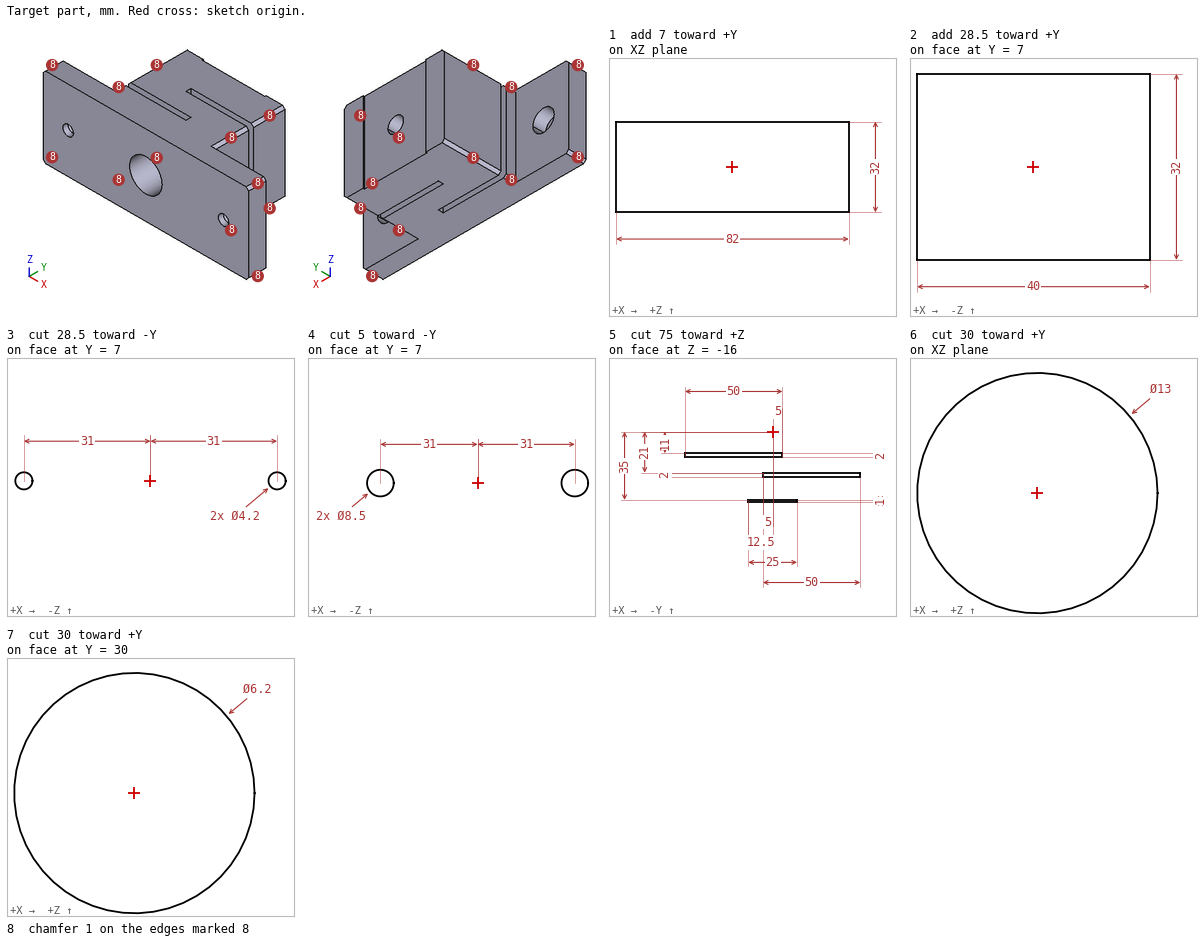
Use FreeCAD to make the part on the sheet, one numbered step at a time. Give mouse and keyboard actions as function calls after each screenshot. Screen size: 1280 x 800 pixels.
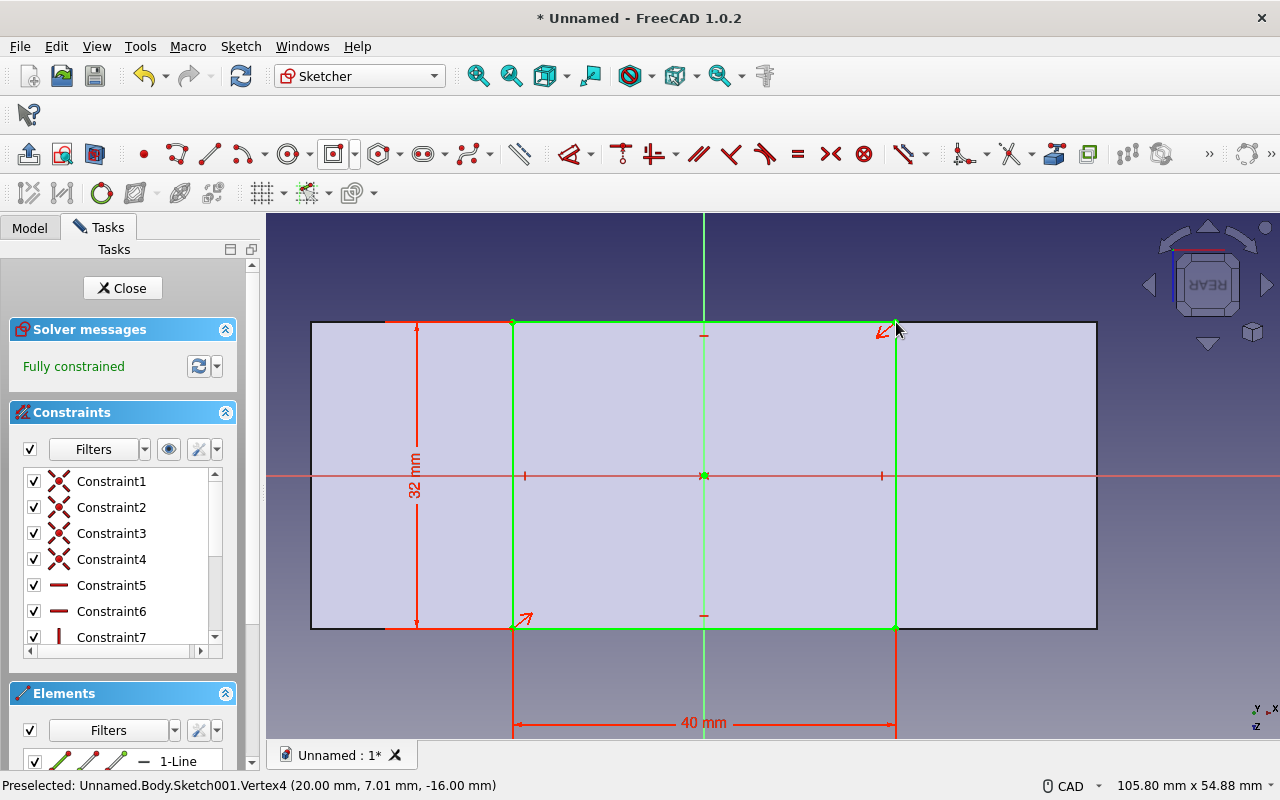
click(123, 288)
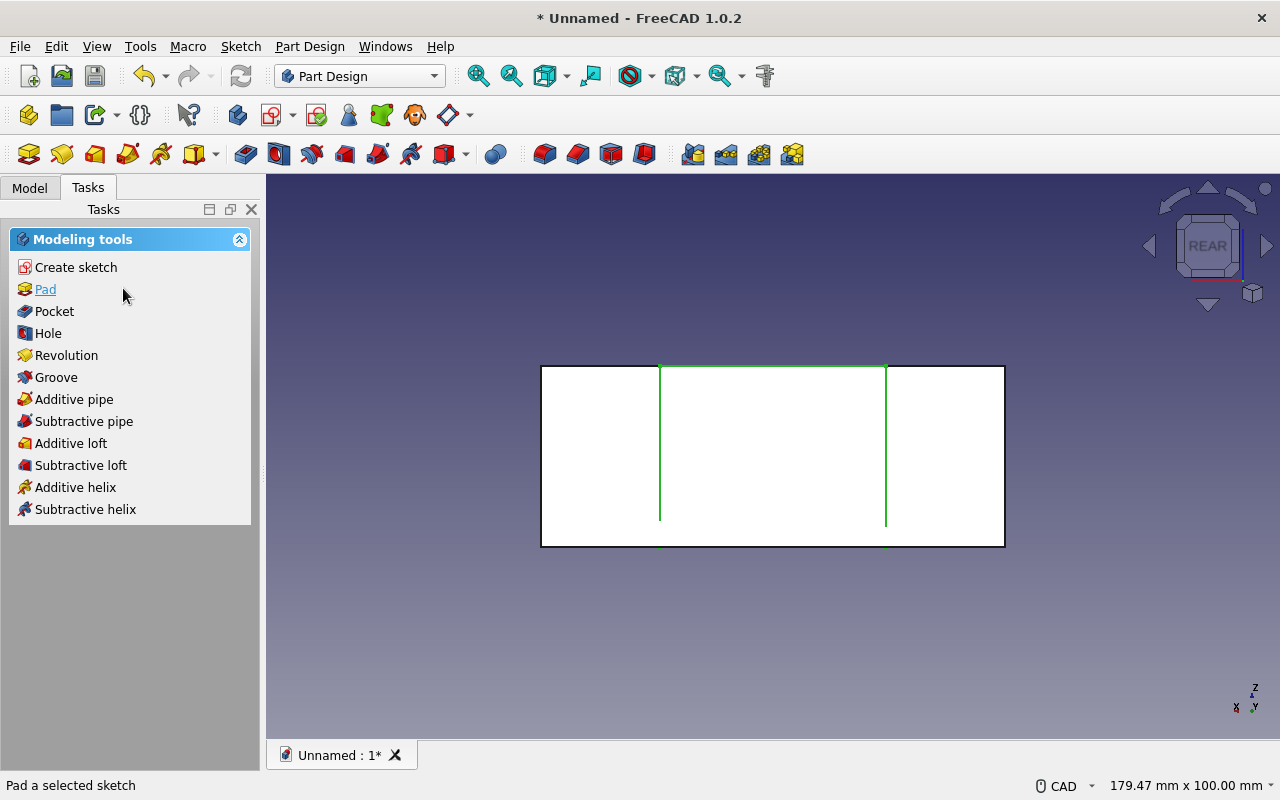
click(29, 154)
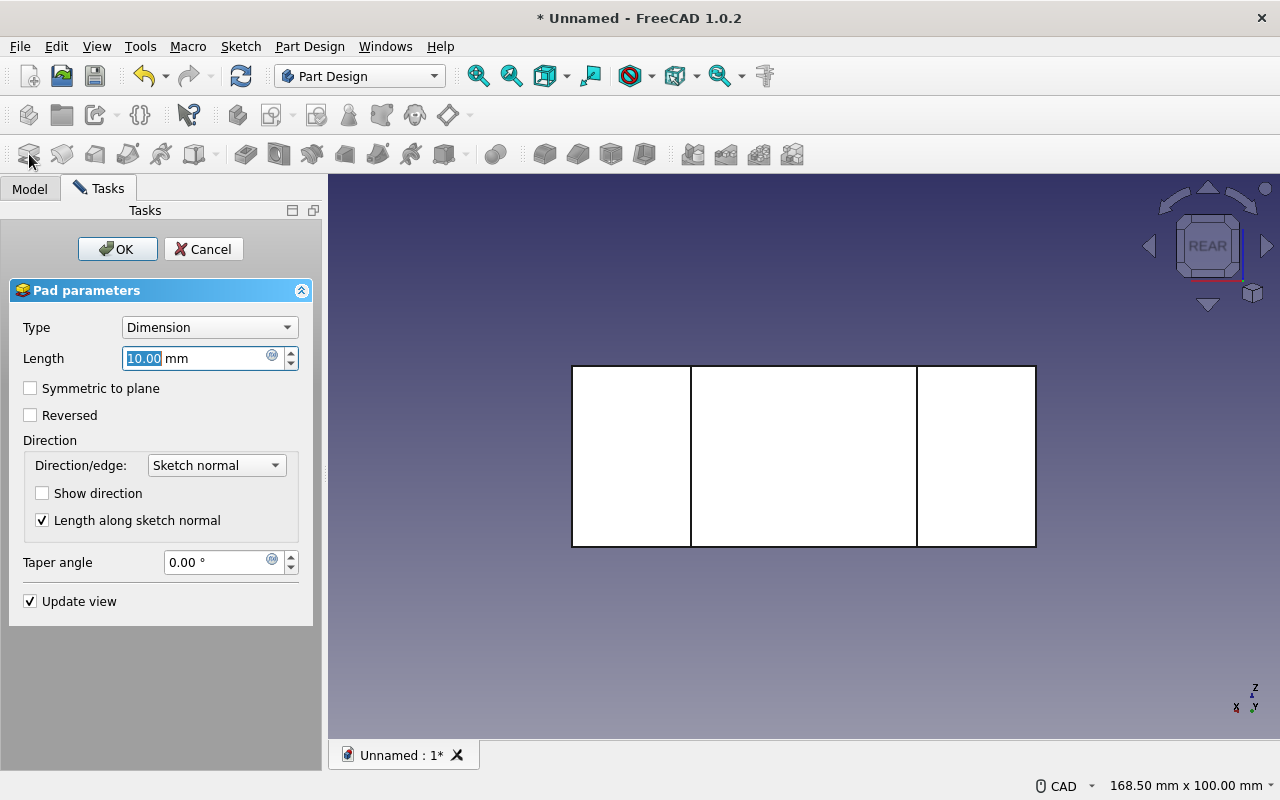
text(28.5)
key(Tab)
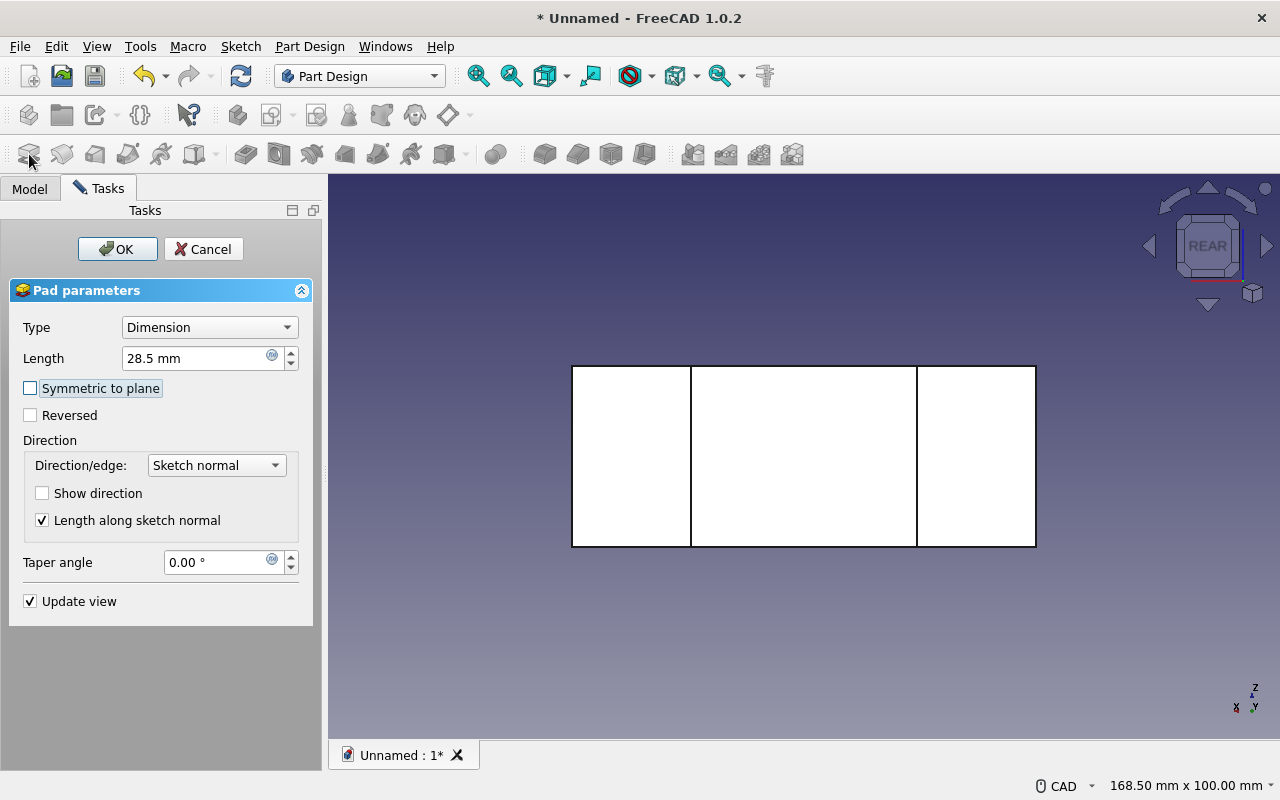
click(118, 249)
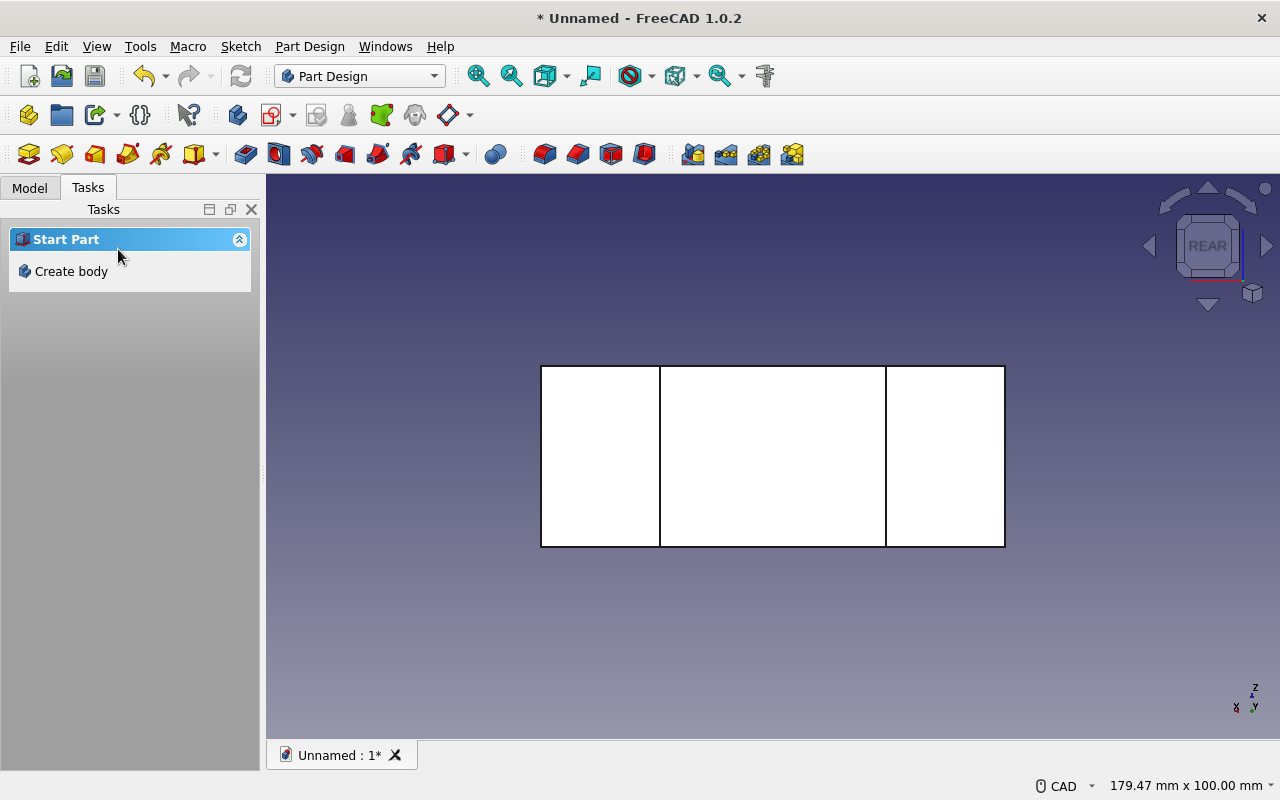
click(601, 430)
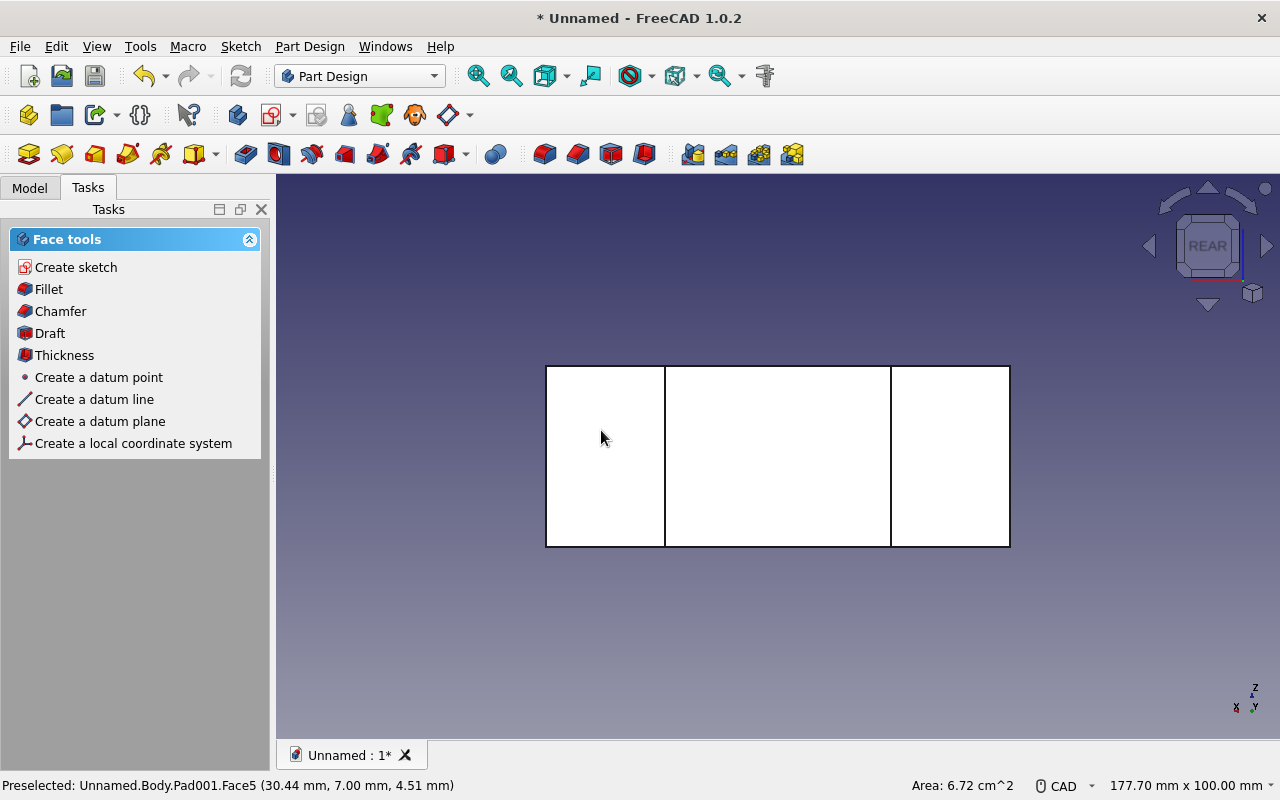
click(270, 116)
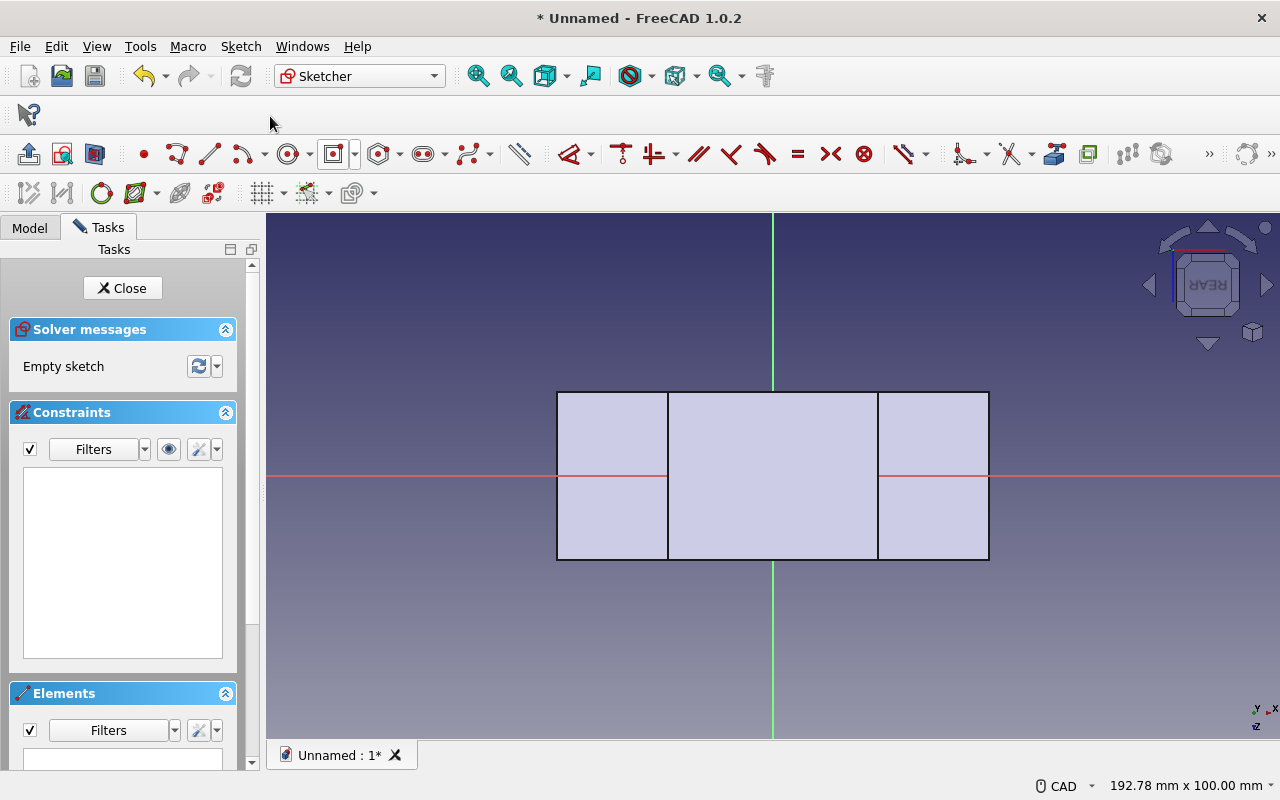
key(q)
key(s)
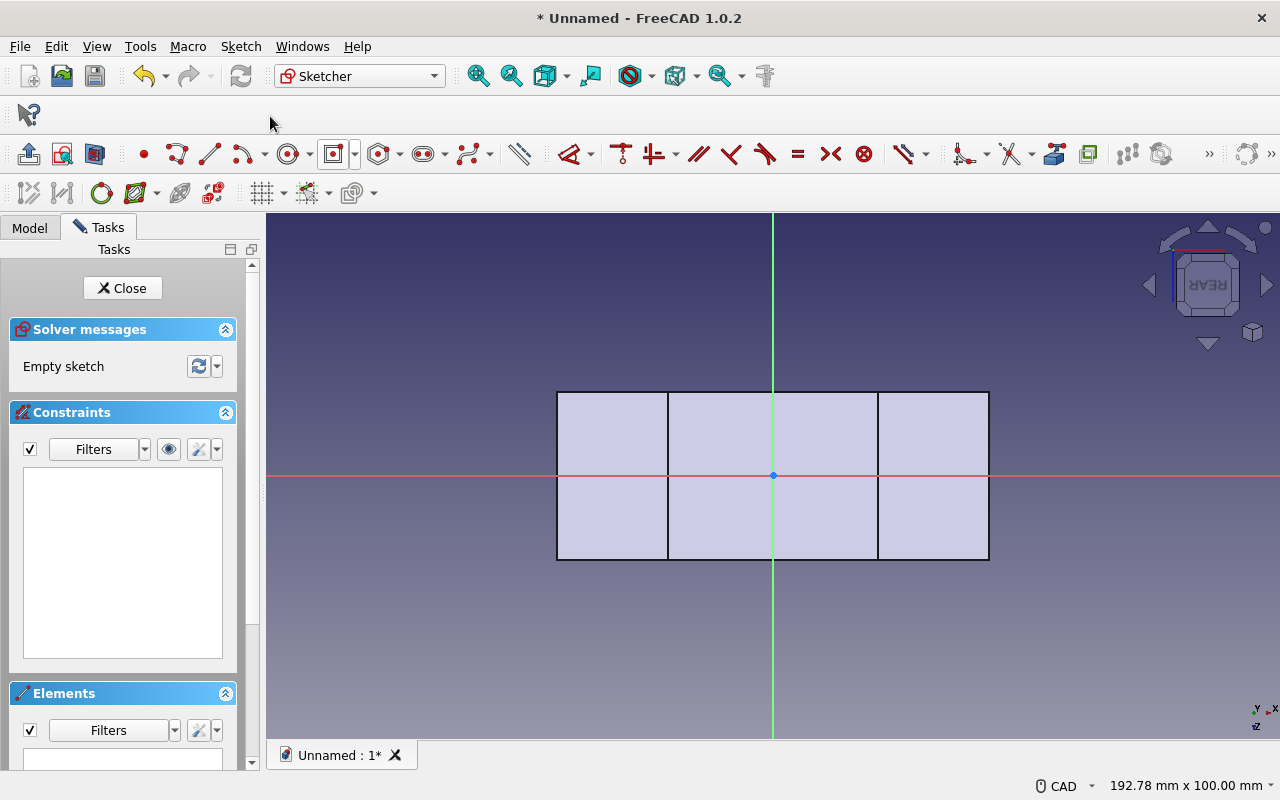
scroll(856, 476, up, 3)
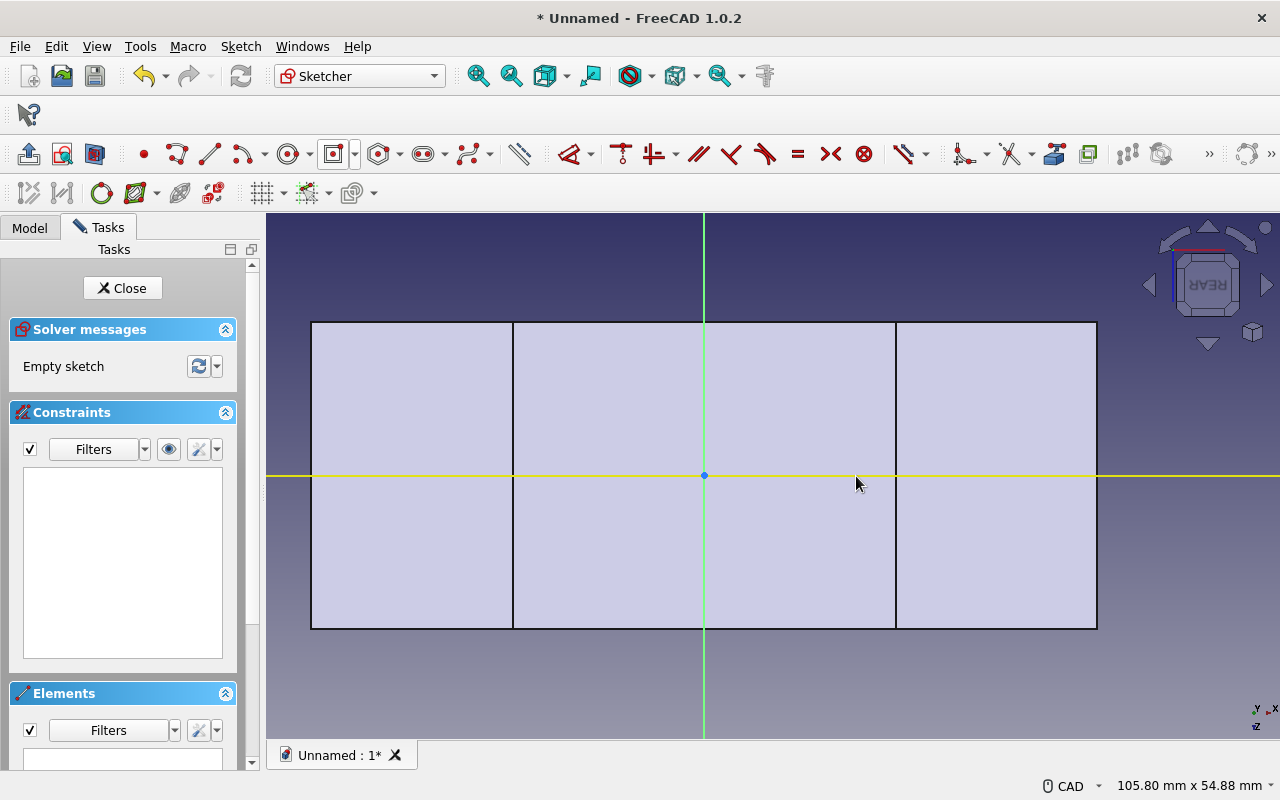
key(g)
key(c)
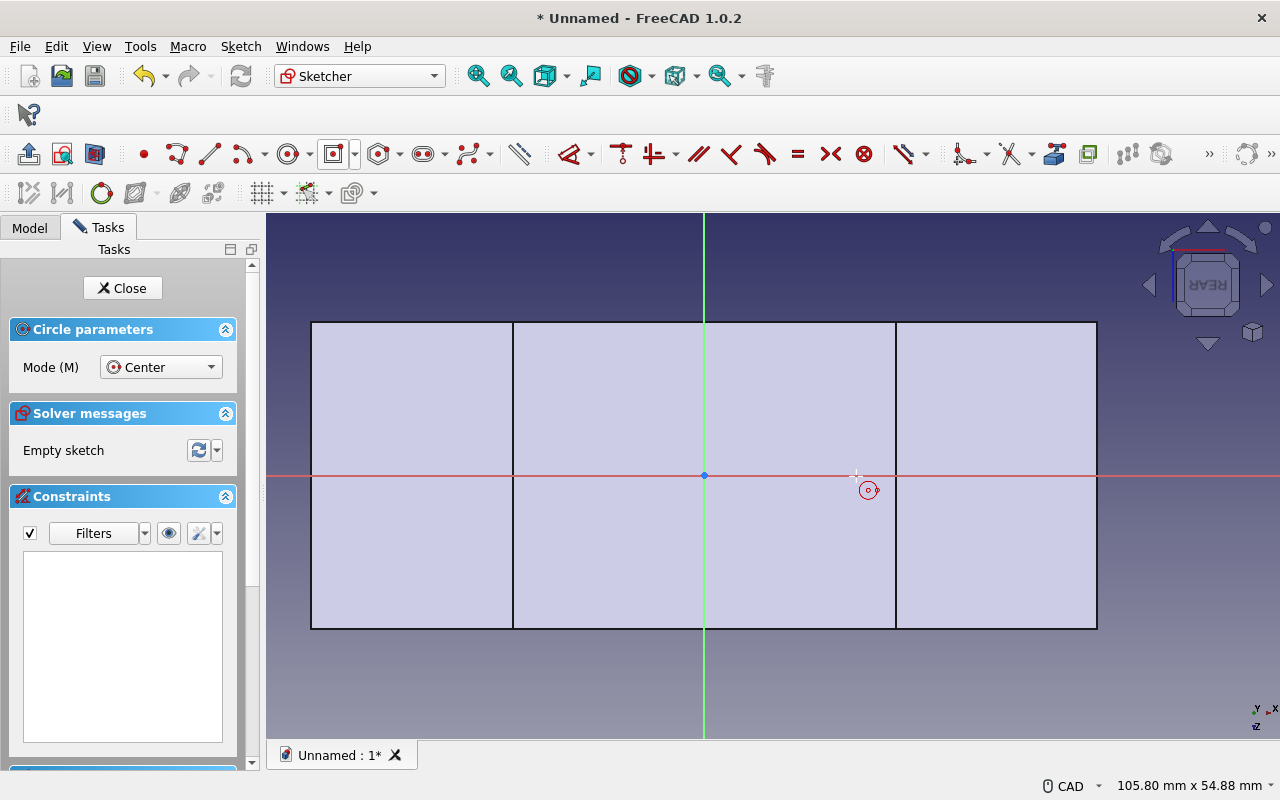
click(1001, 476)
move(1016, 461)